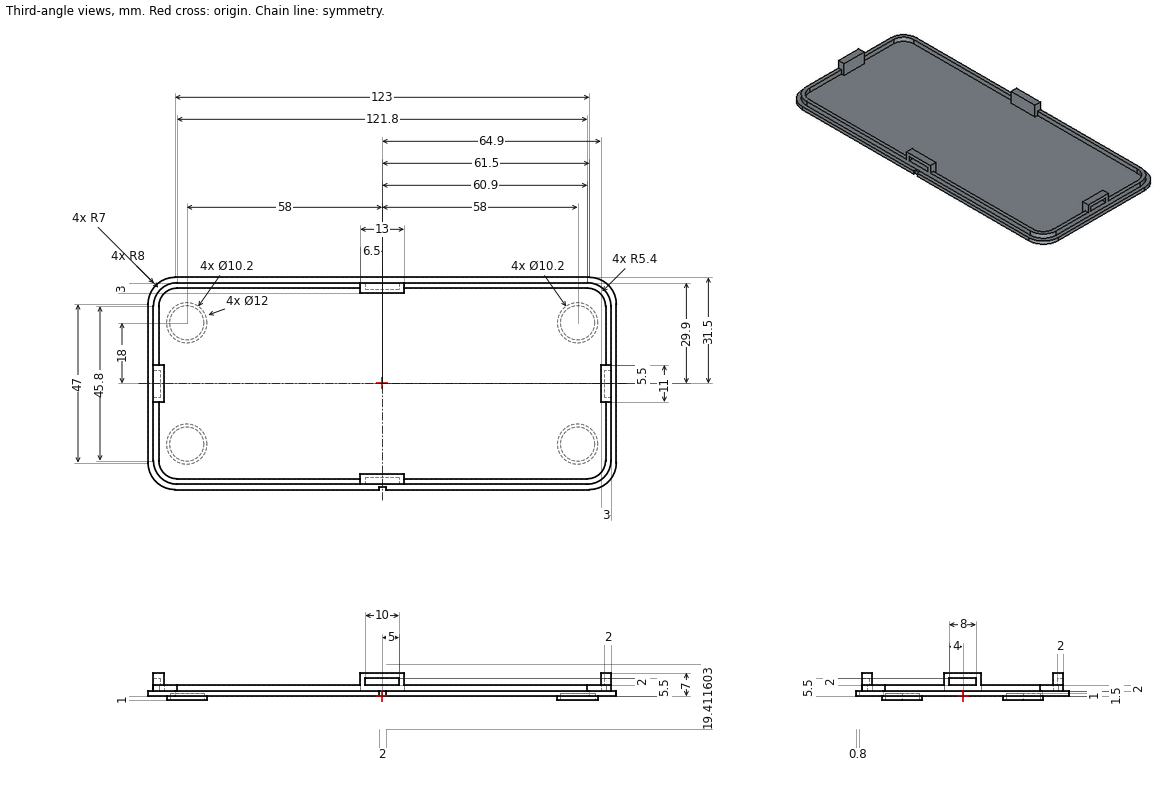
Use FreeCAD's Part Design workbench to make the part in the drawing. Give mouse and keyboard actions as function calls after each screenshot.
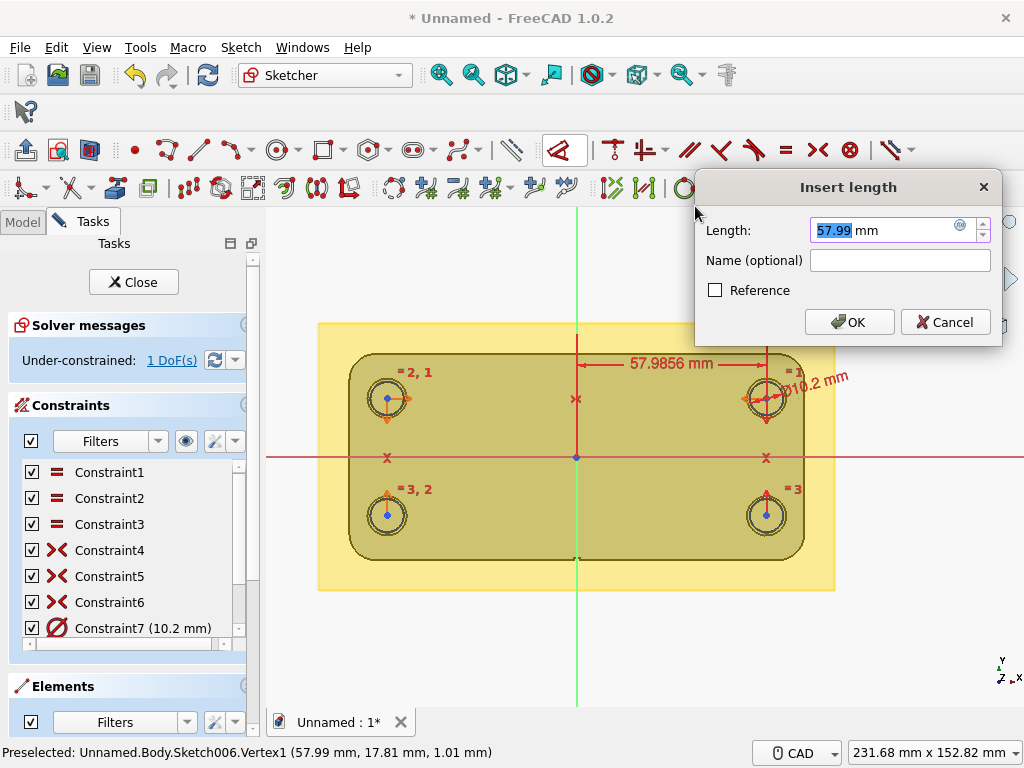
text(58)
key(Return)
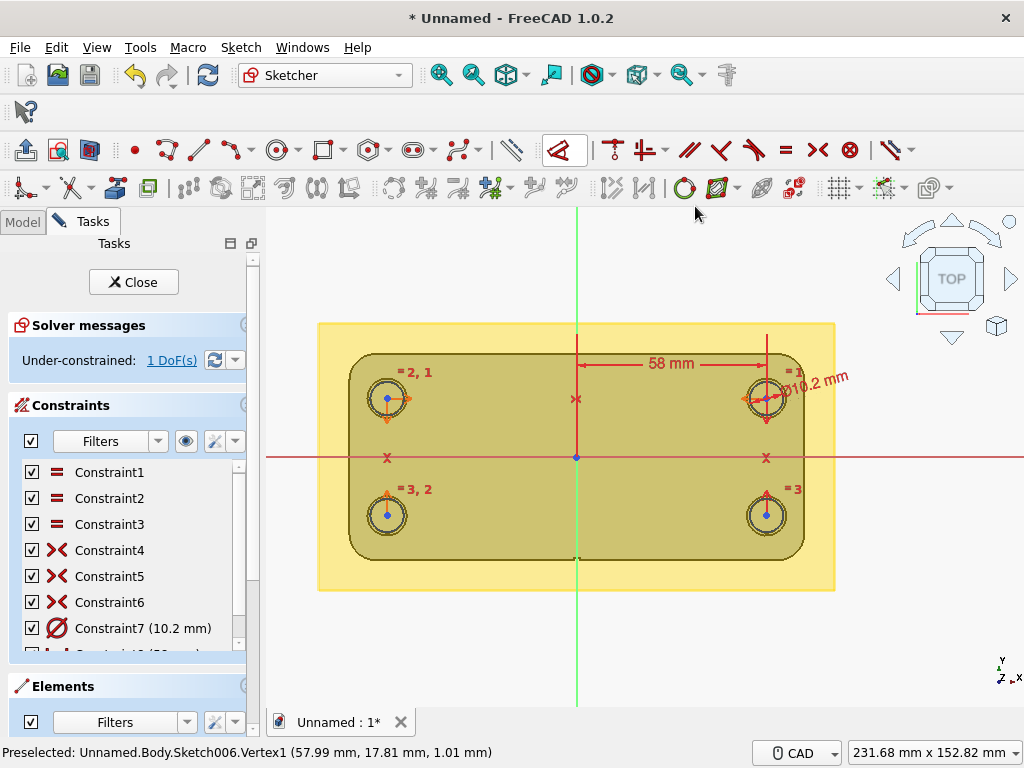
click(767, 399)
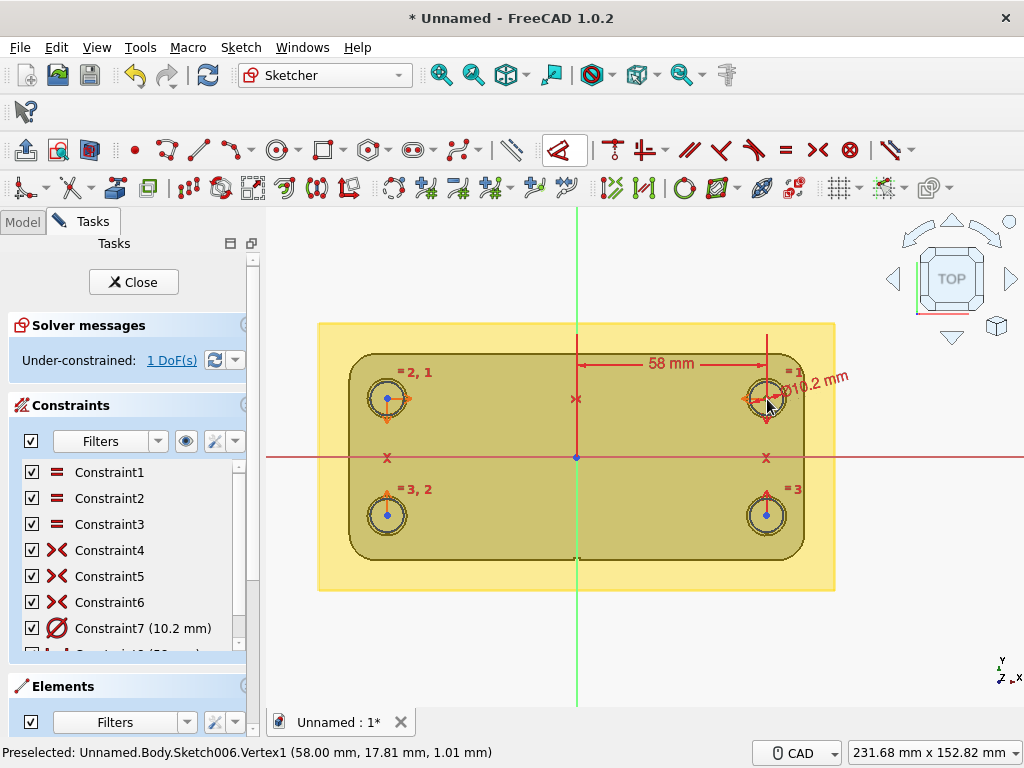
click(582, 150)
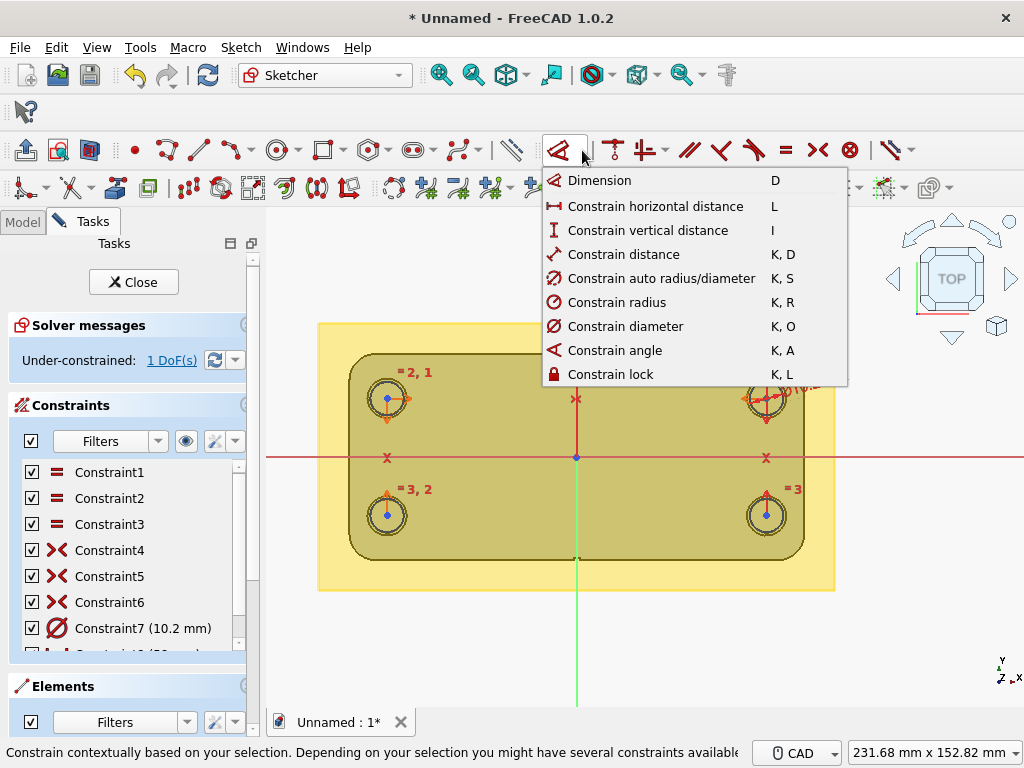
click(695, 230)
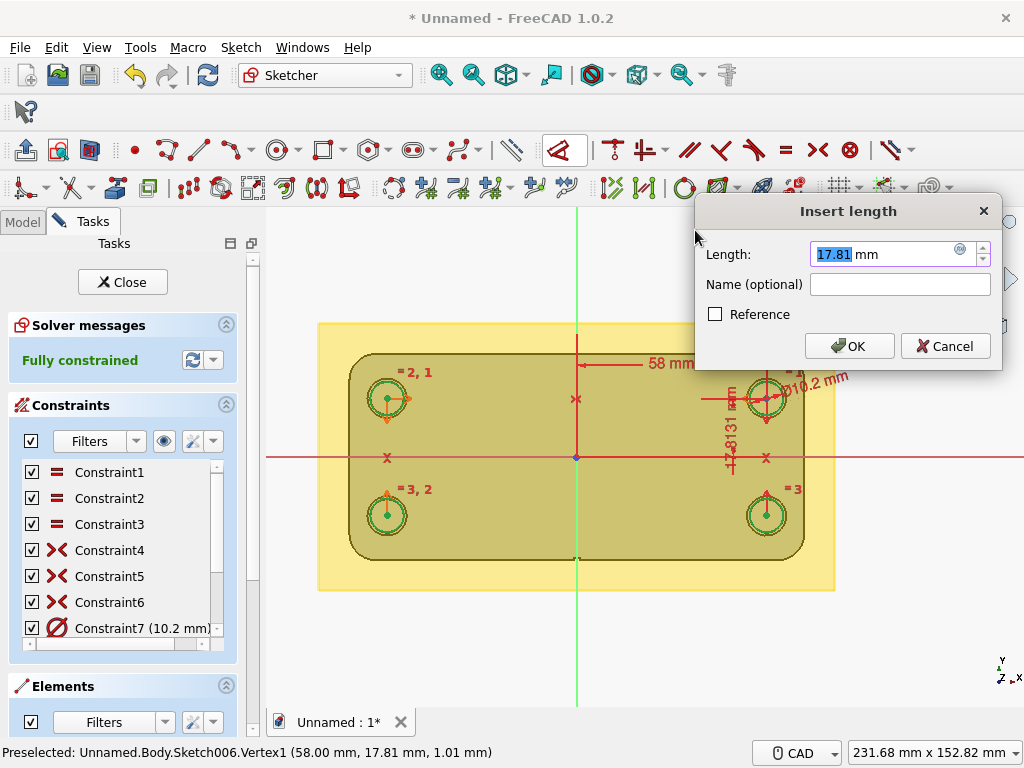
text(18)
key(Return)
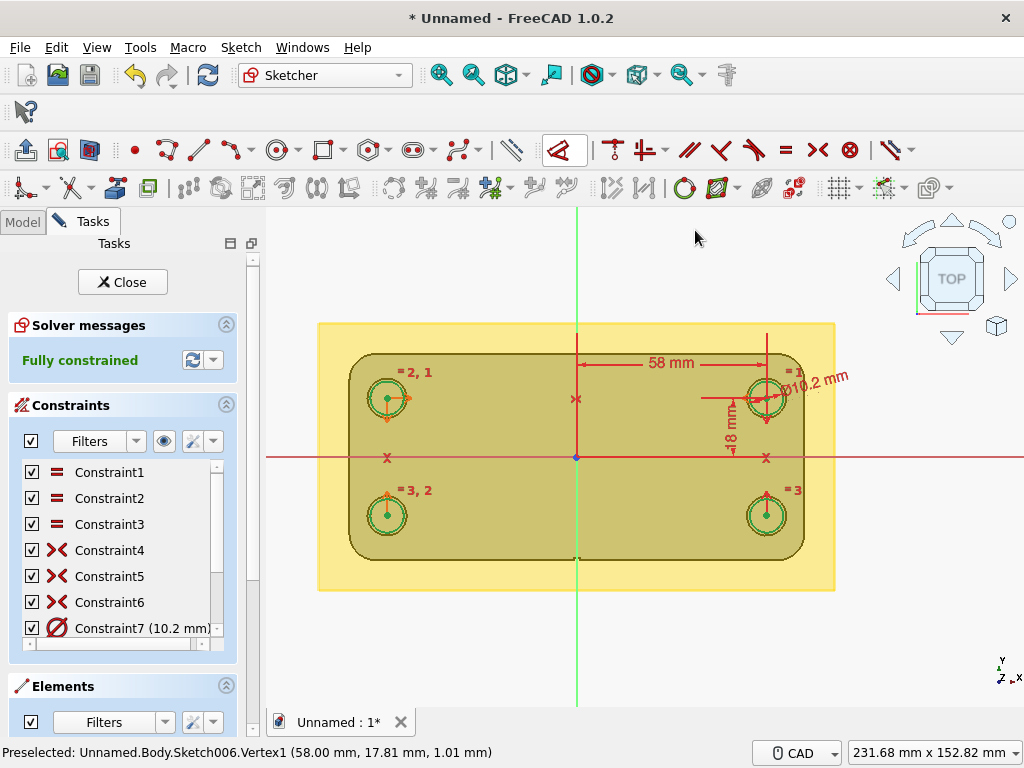
click(123, 282)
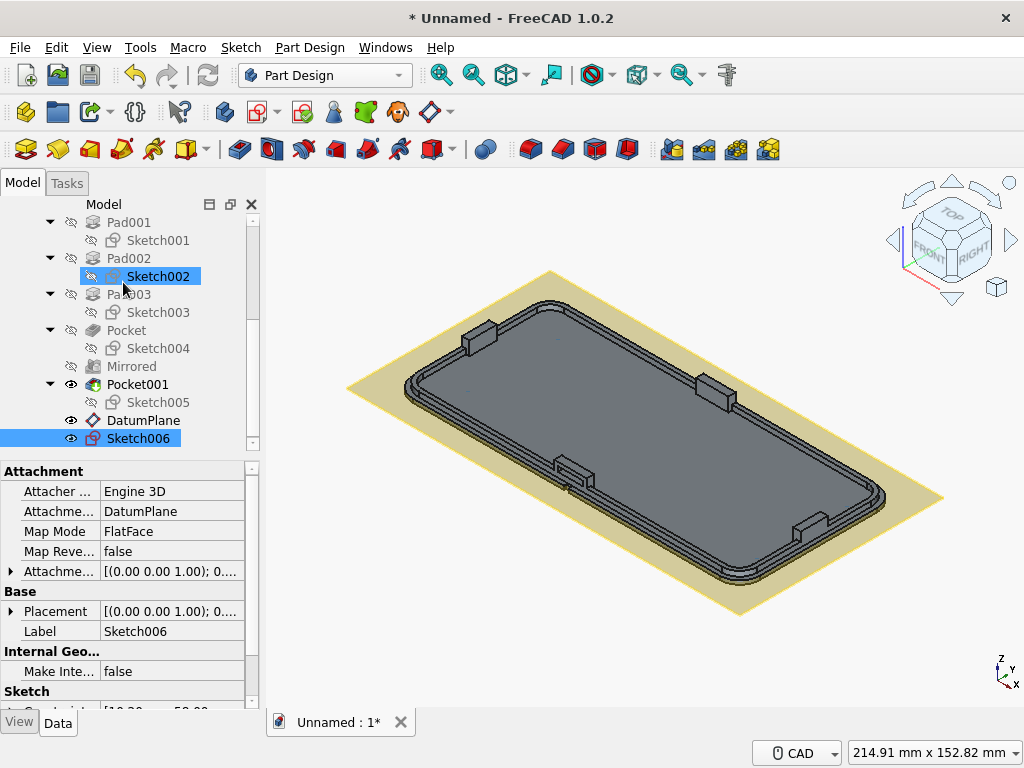
click(240, 150)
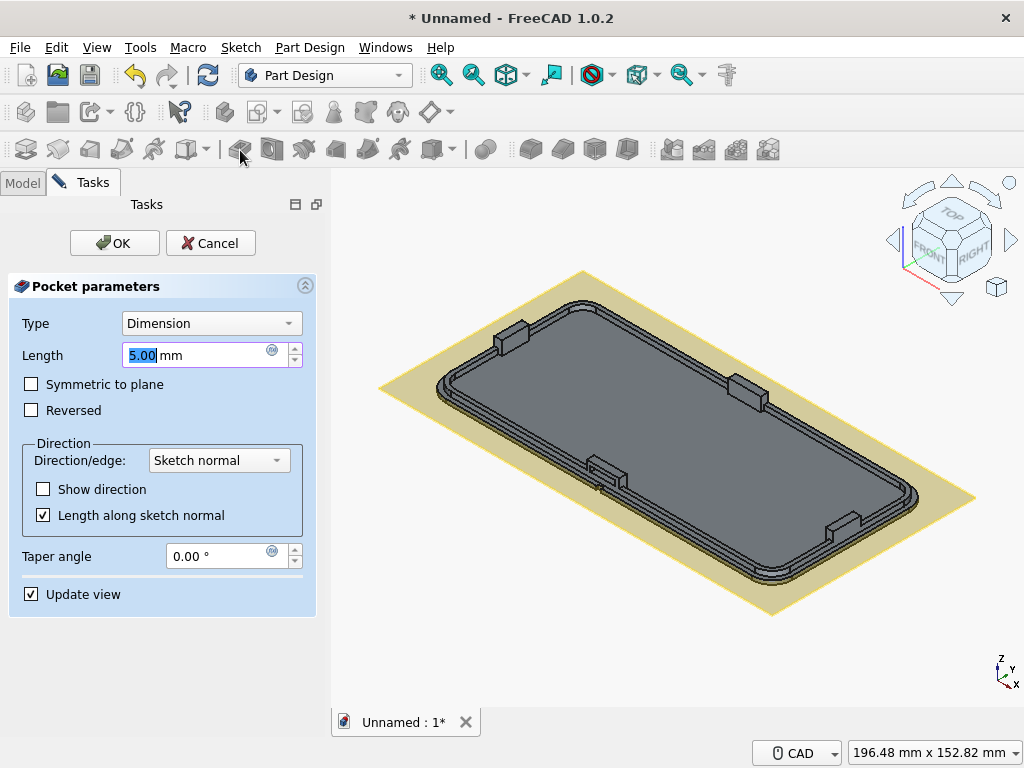
text(1)
key(Tab)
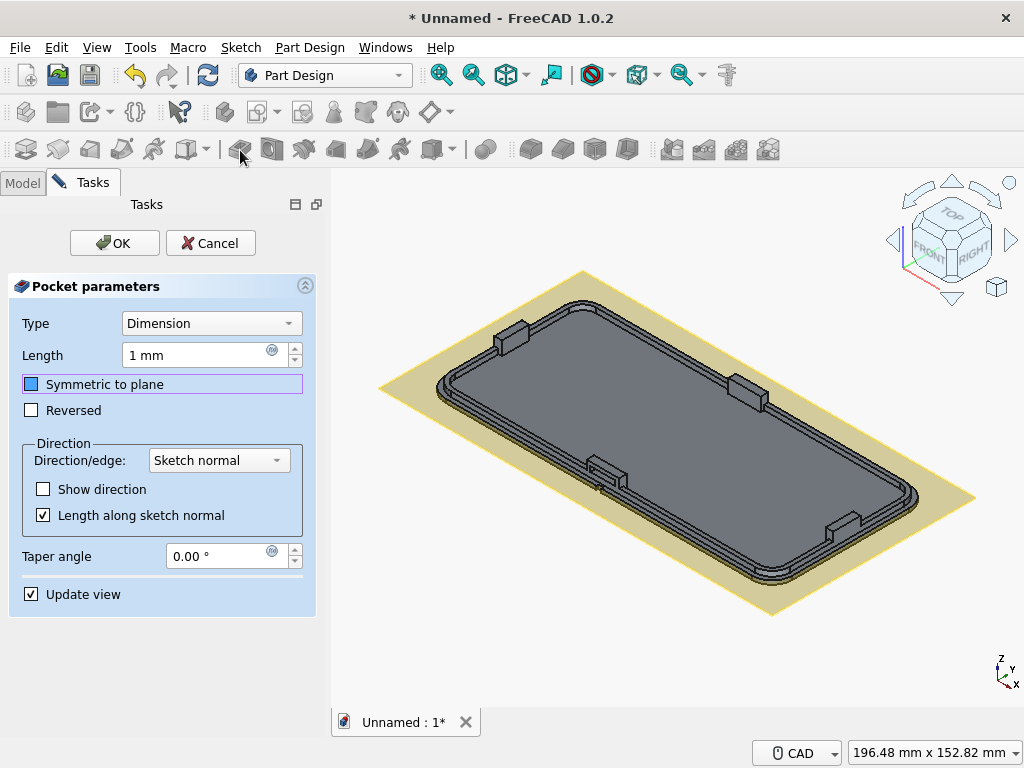
click(115, 243)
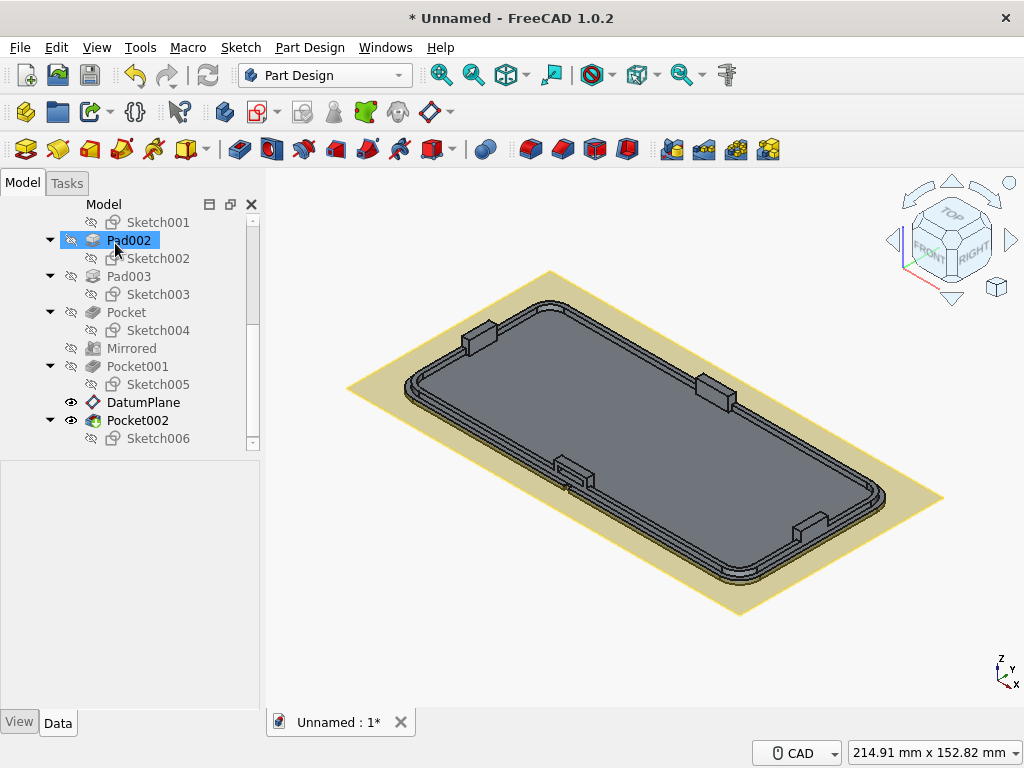
click(116, 402)
key(space)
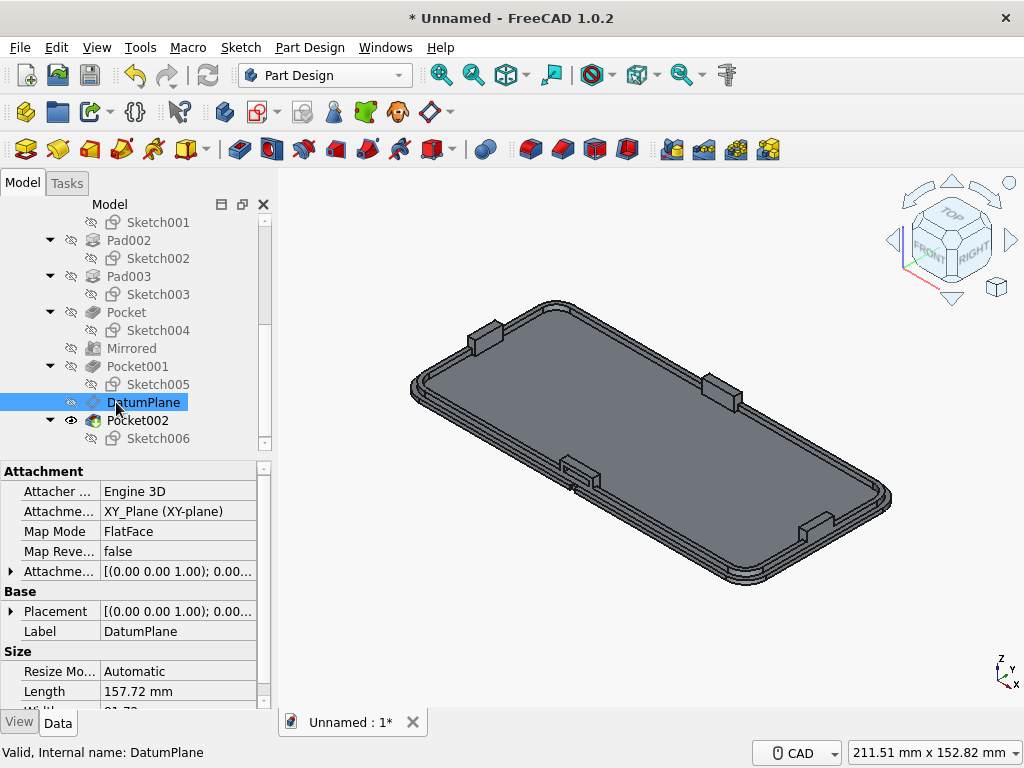
key(3)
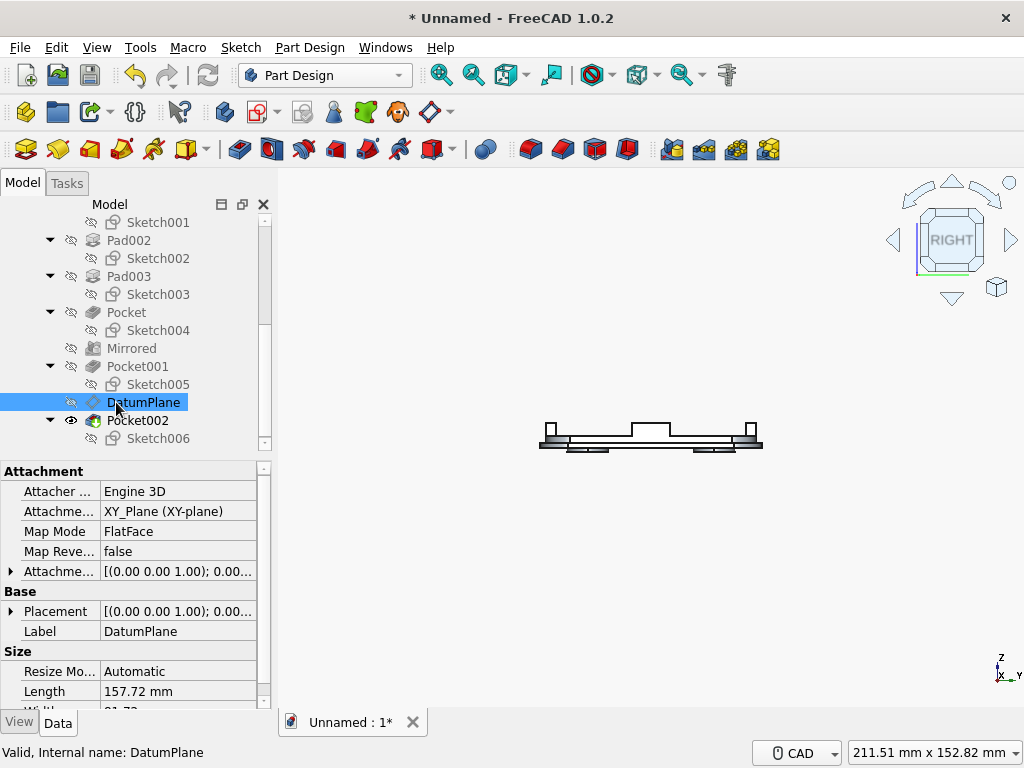
click(442, 76)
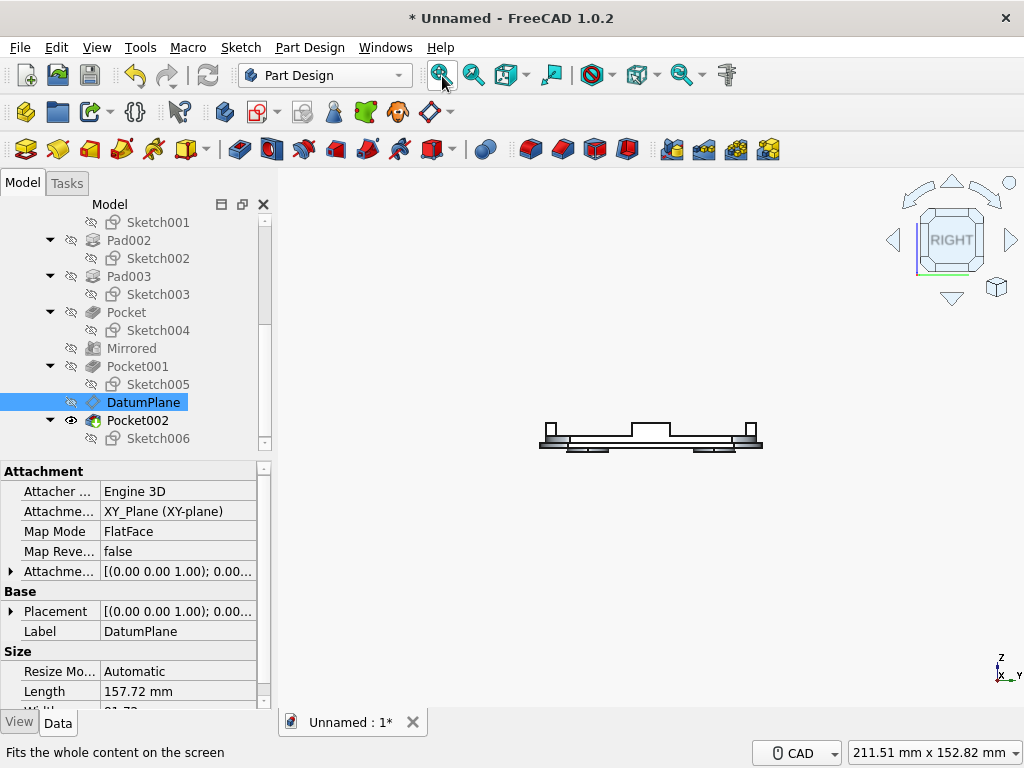
click(651, 432)